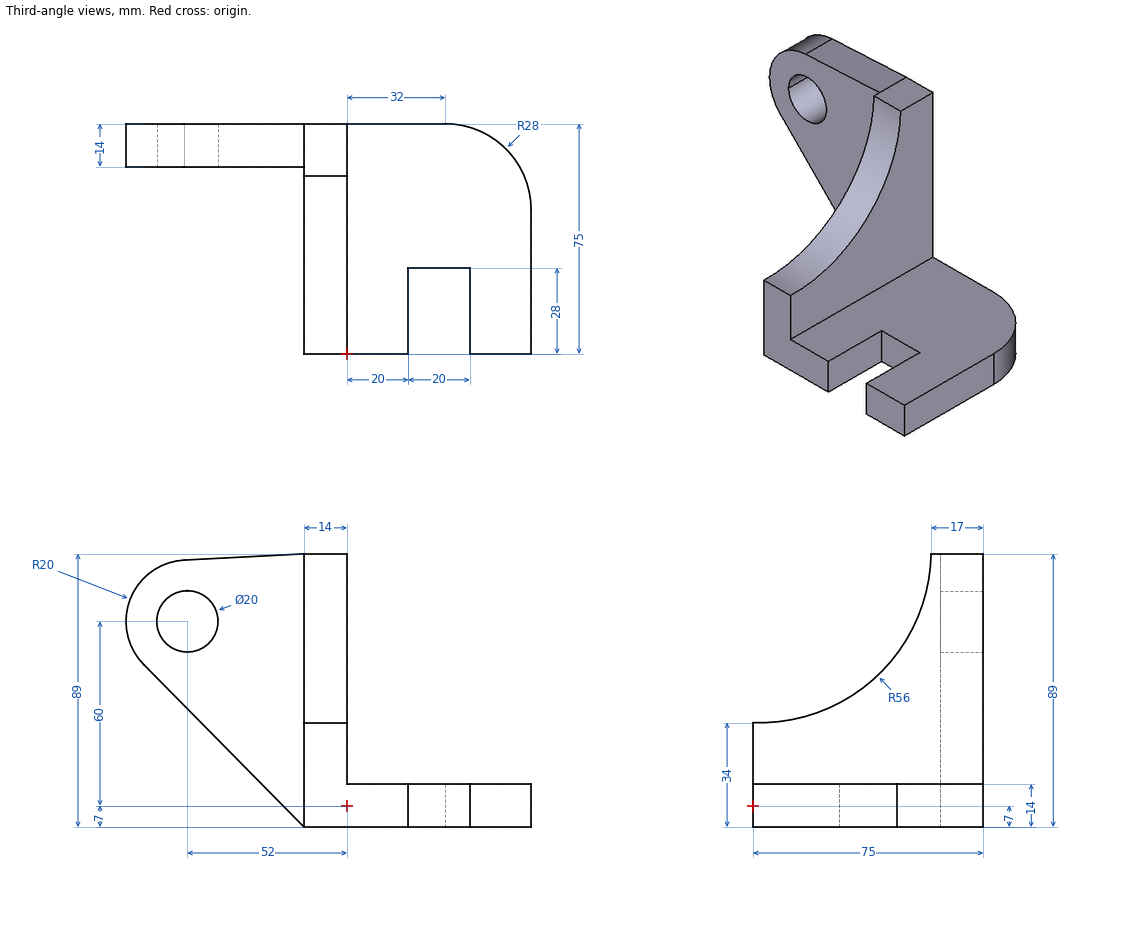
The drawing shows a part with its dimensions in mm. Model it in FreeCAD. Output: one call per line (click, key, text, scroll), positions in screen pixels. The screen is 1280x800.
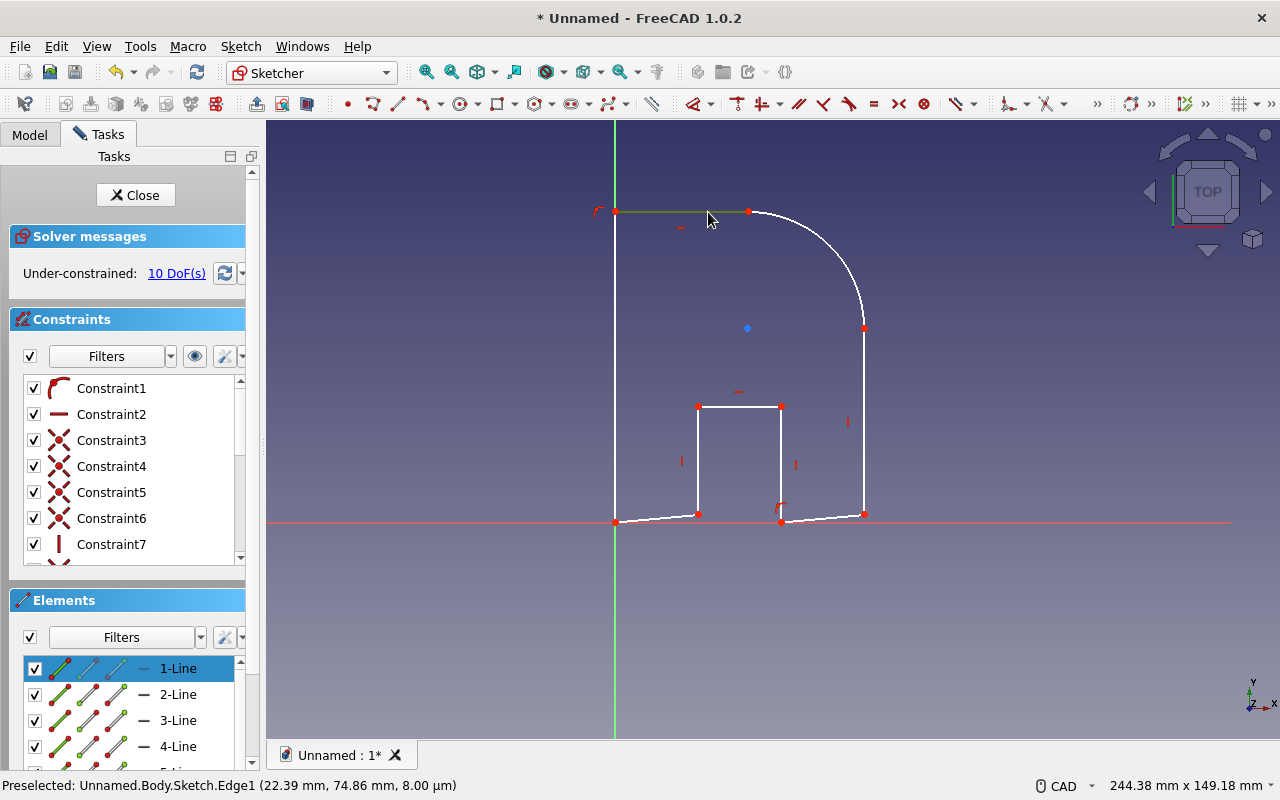
click(852, 276)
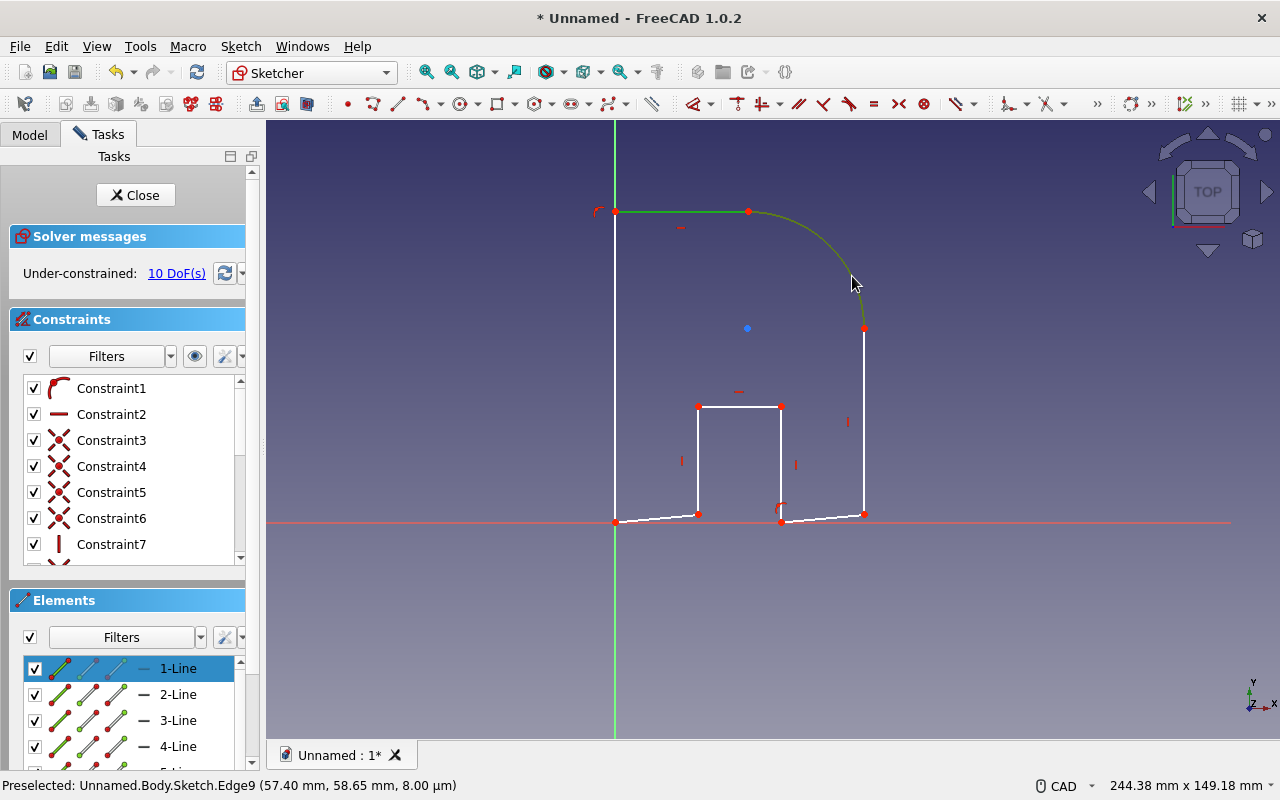
click(849, 104)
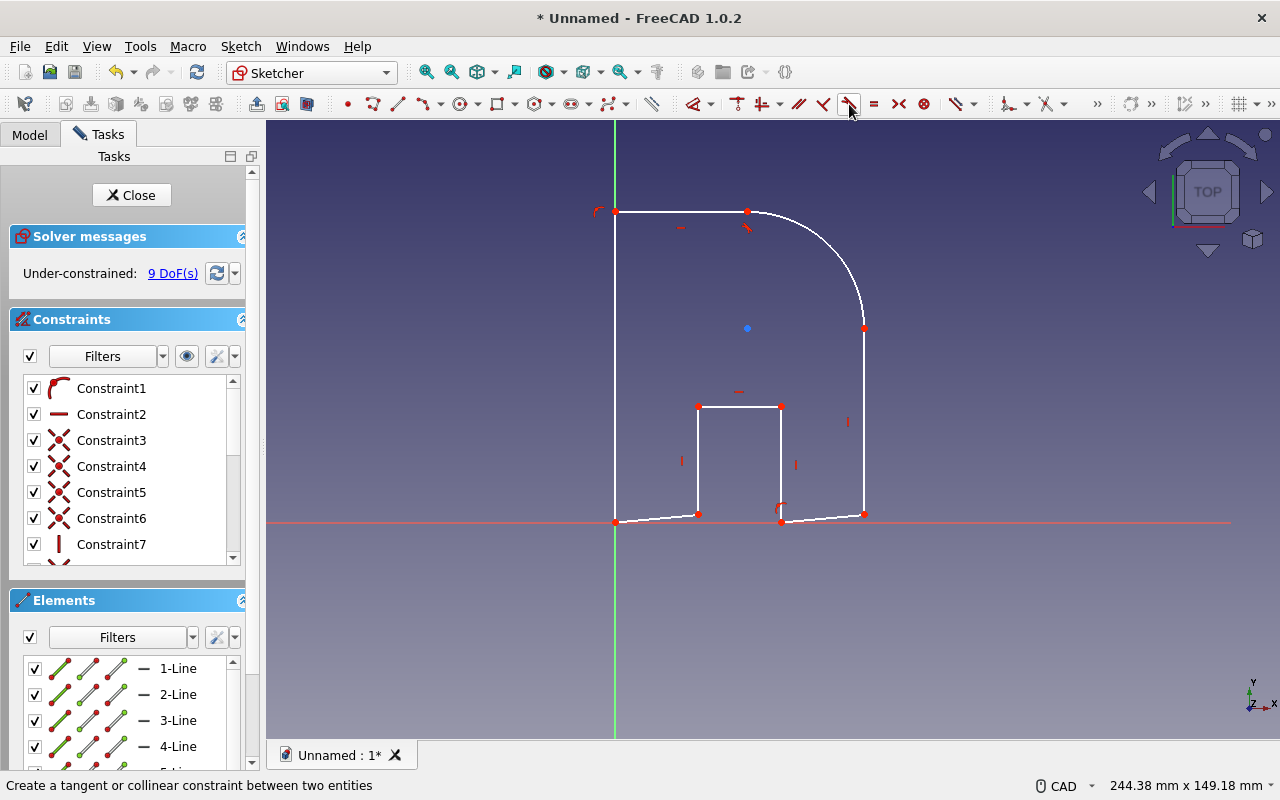
click(864, 459)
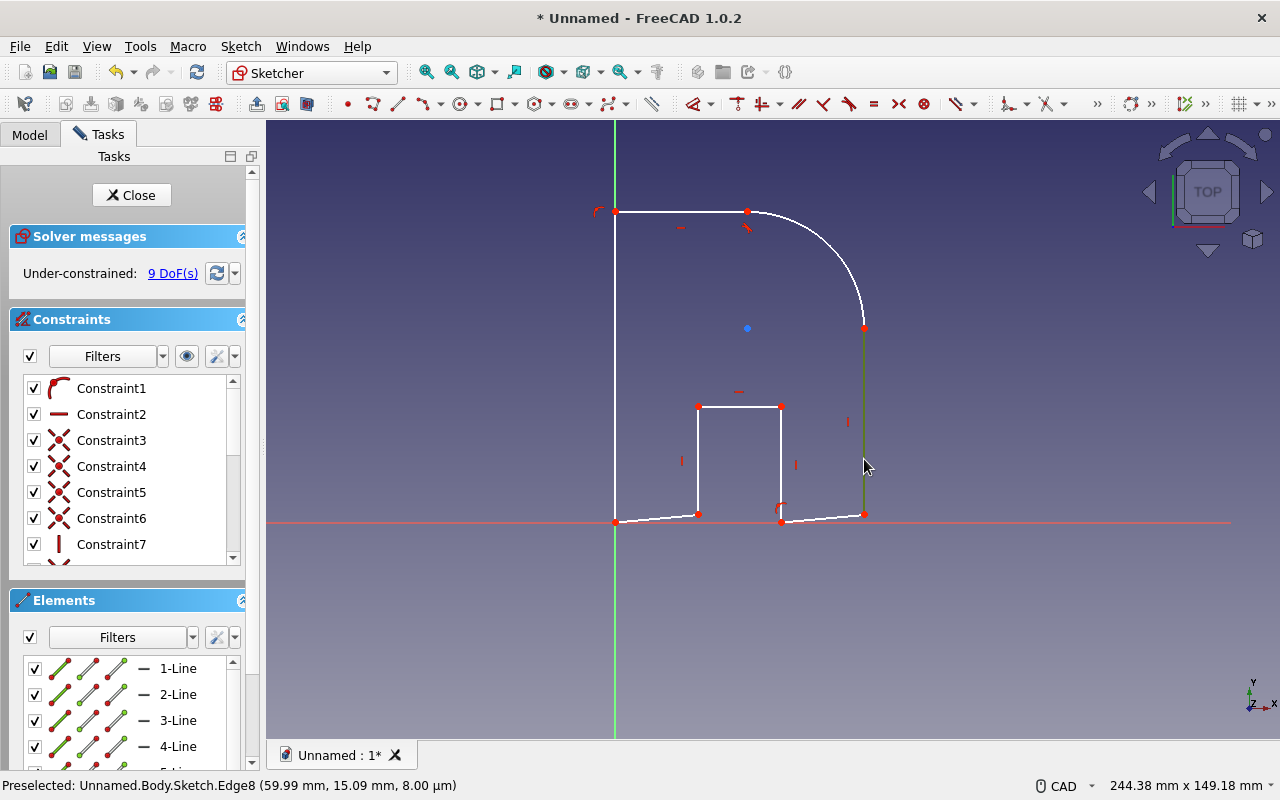
click(852, 276)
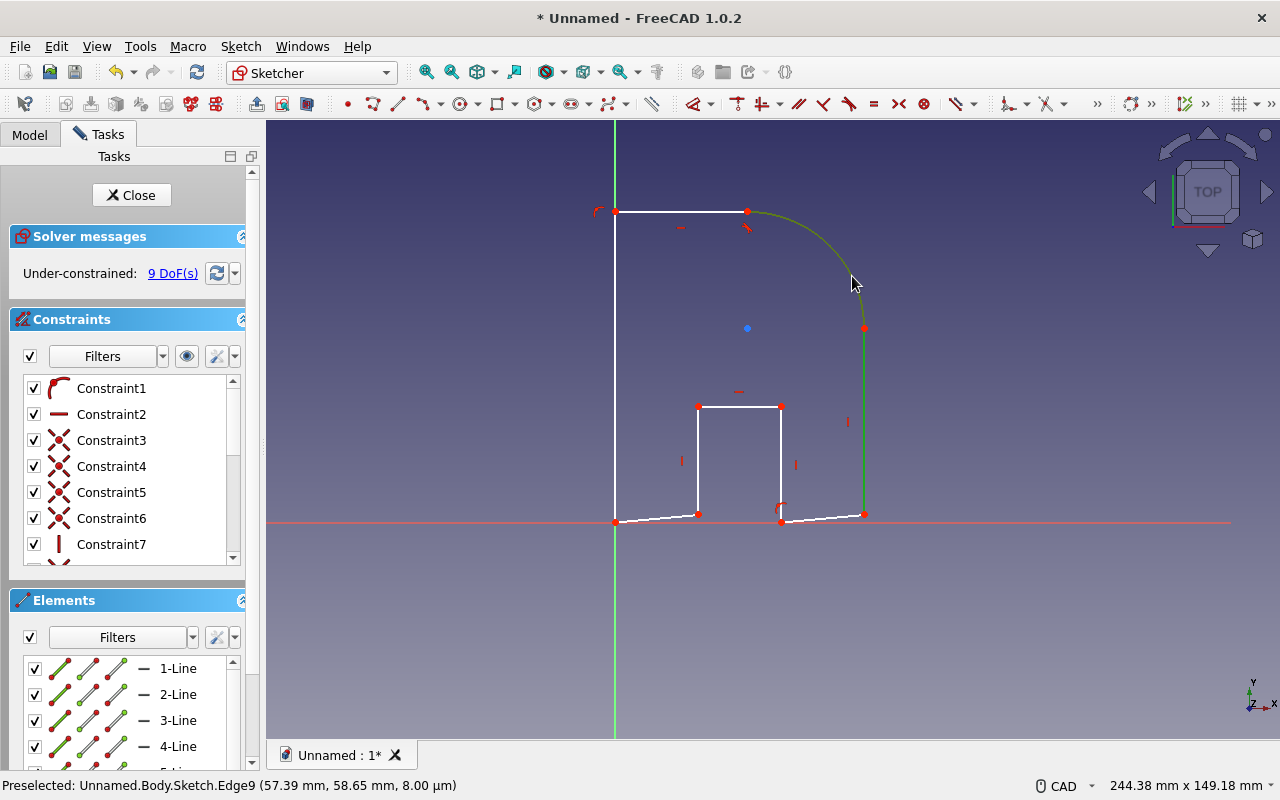
click(849, 104)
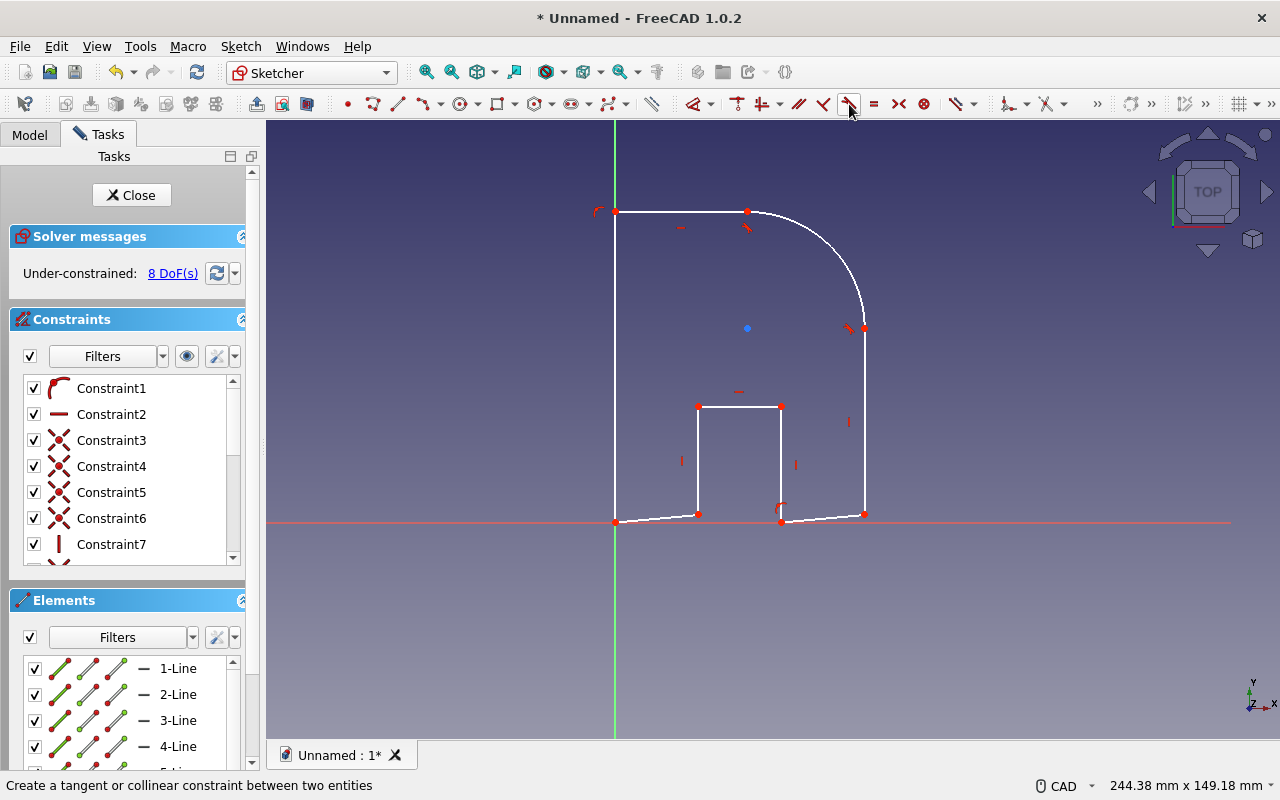
click(640, 520)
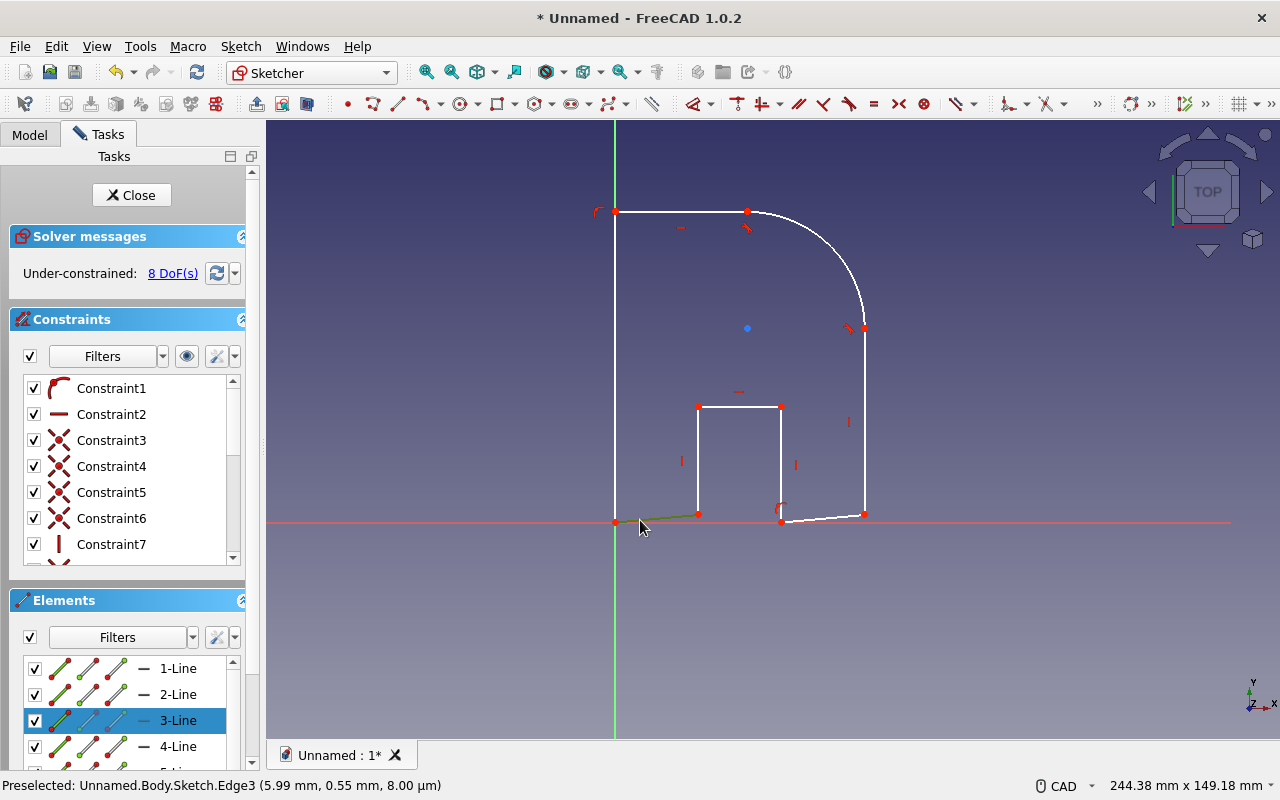
key(h)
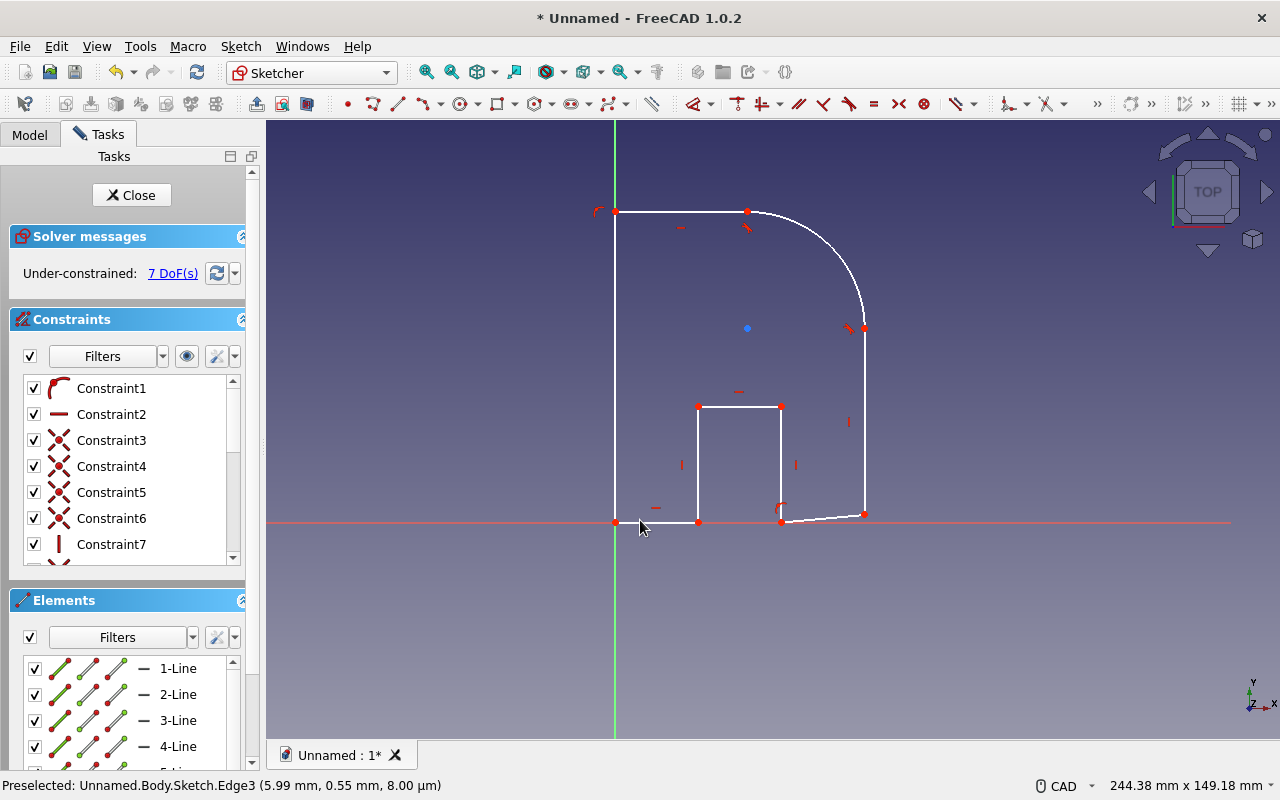
click(806, 520)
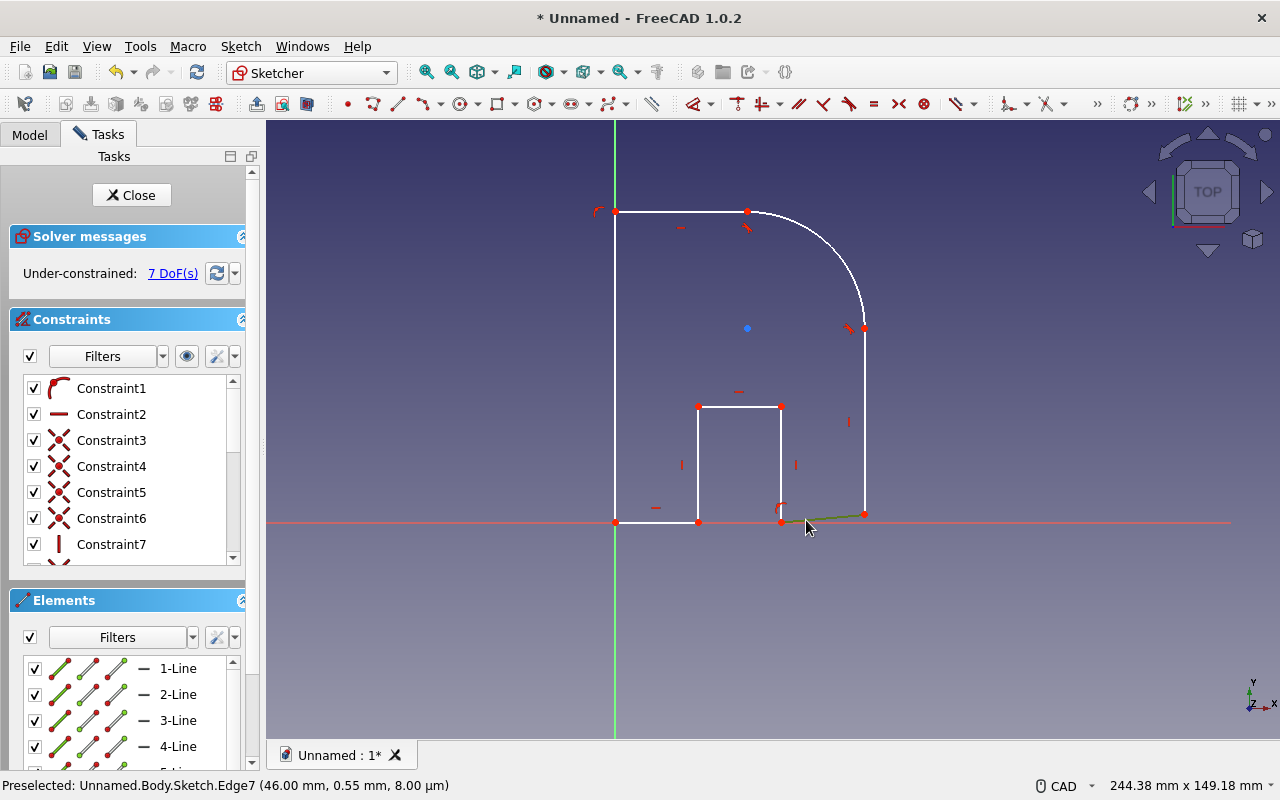
key(h)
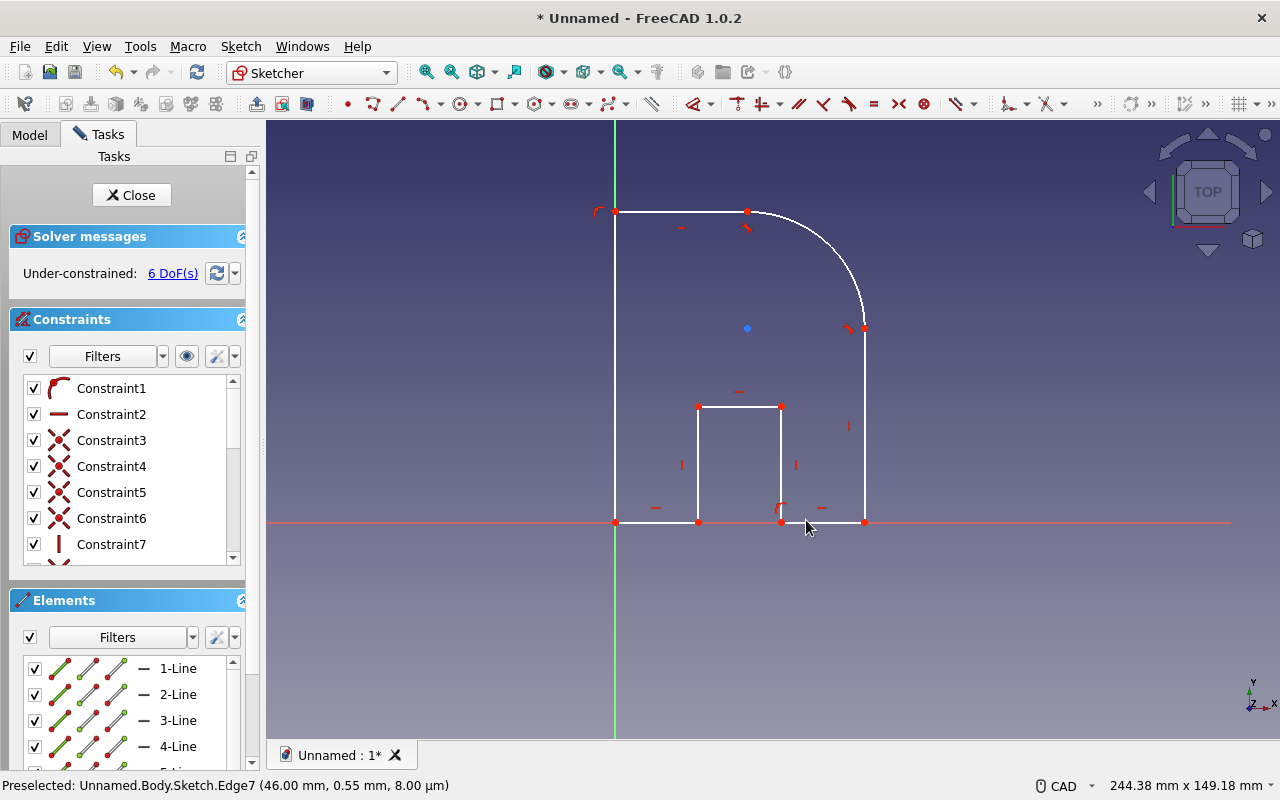
click(692, 104)